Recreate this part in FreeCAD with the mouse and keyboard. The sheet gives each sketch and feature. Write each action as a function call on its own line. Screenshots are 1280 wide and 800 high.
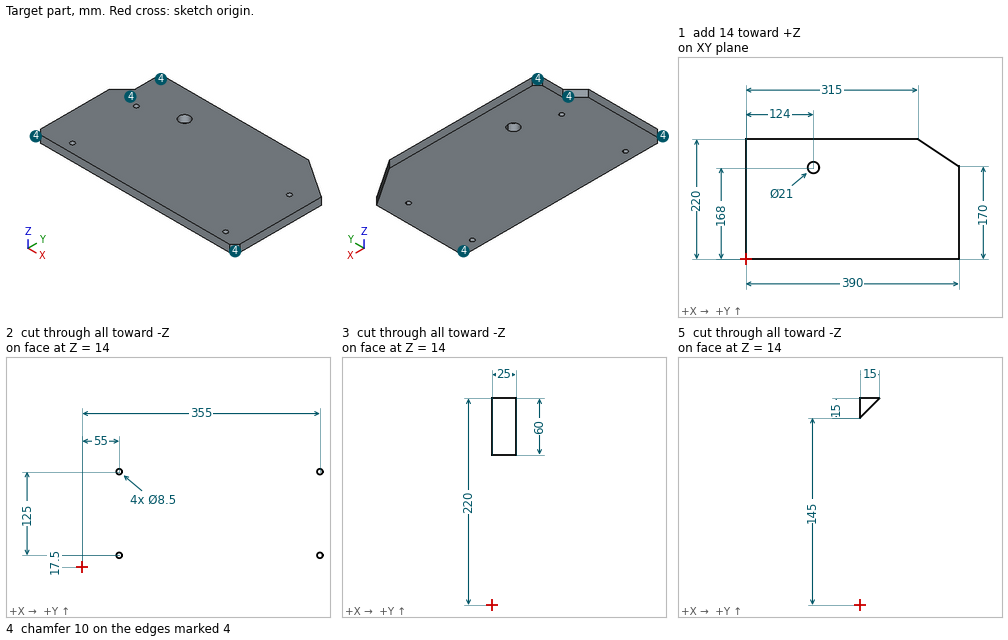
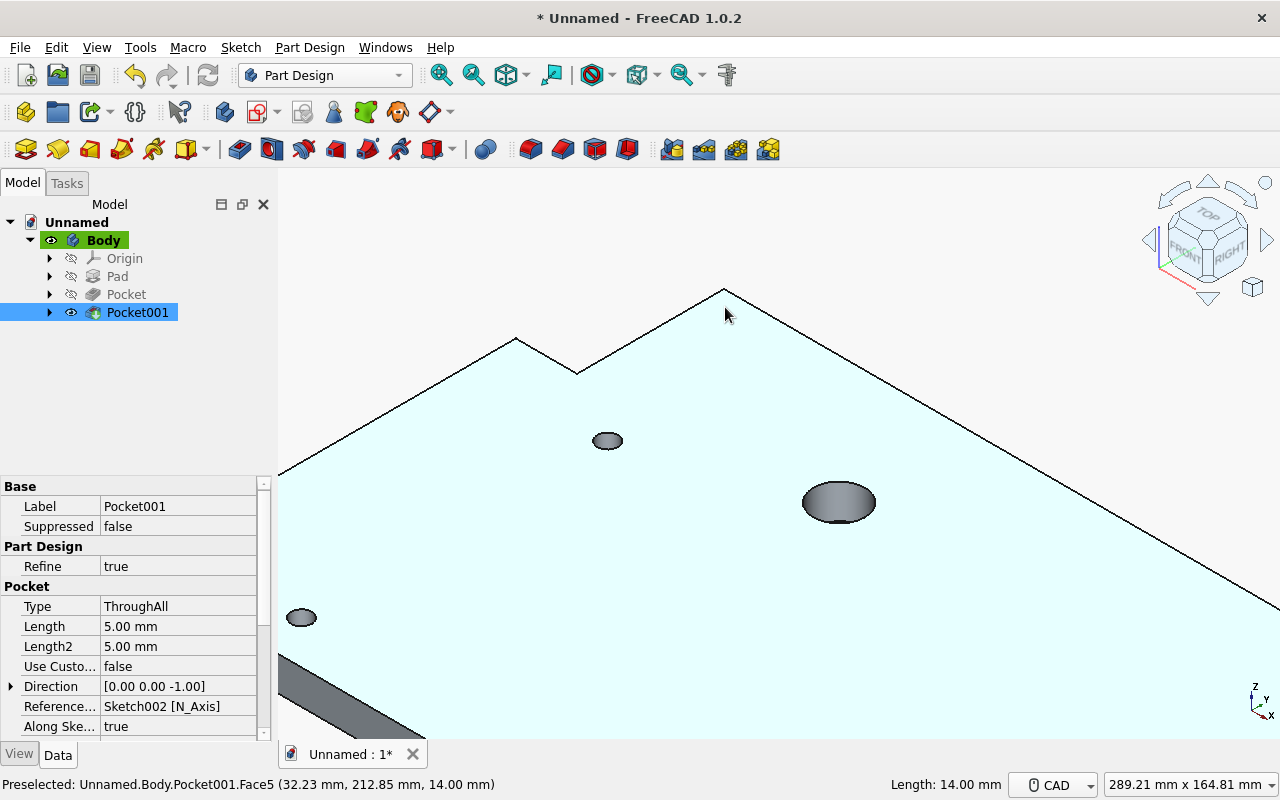
key(v)
key(f)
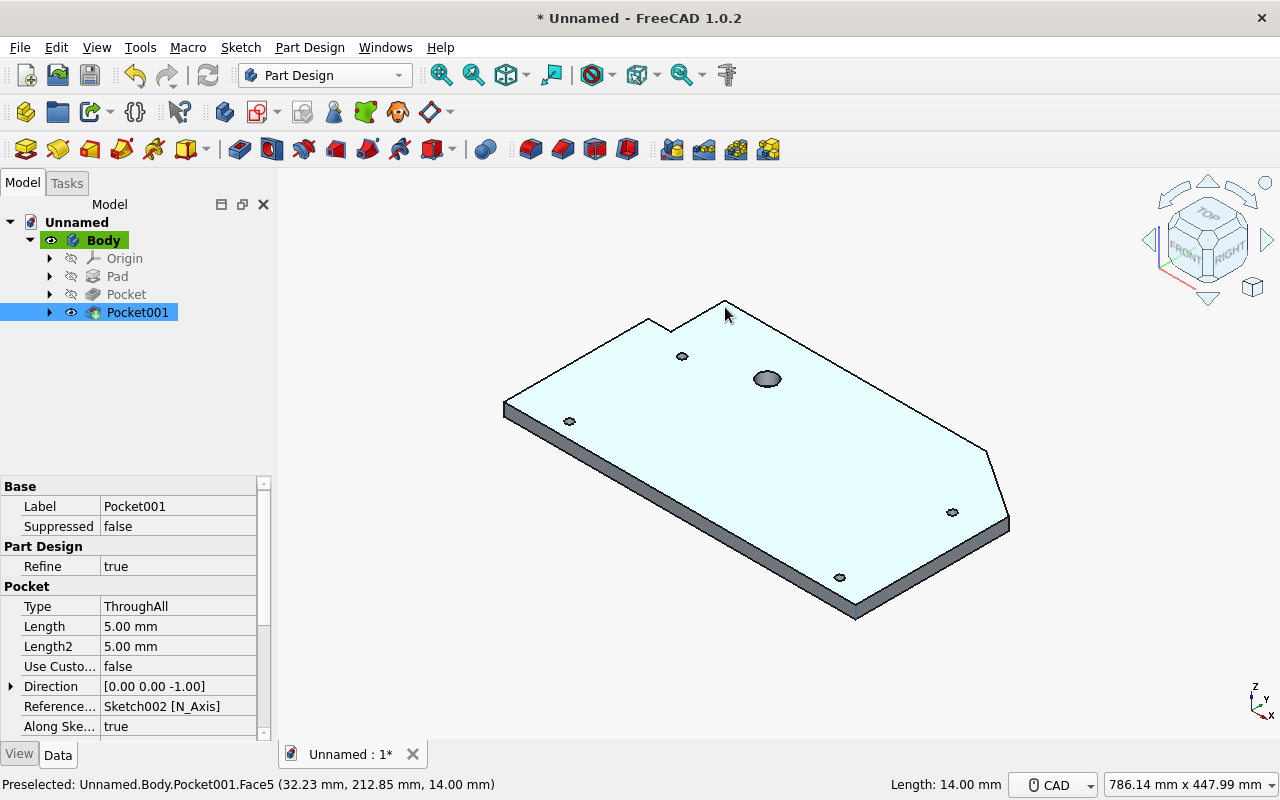
key(2)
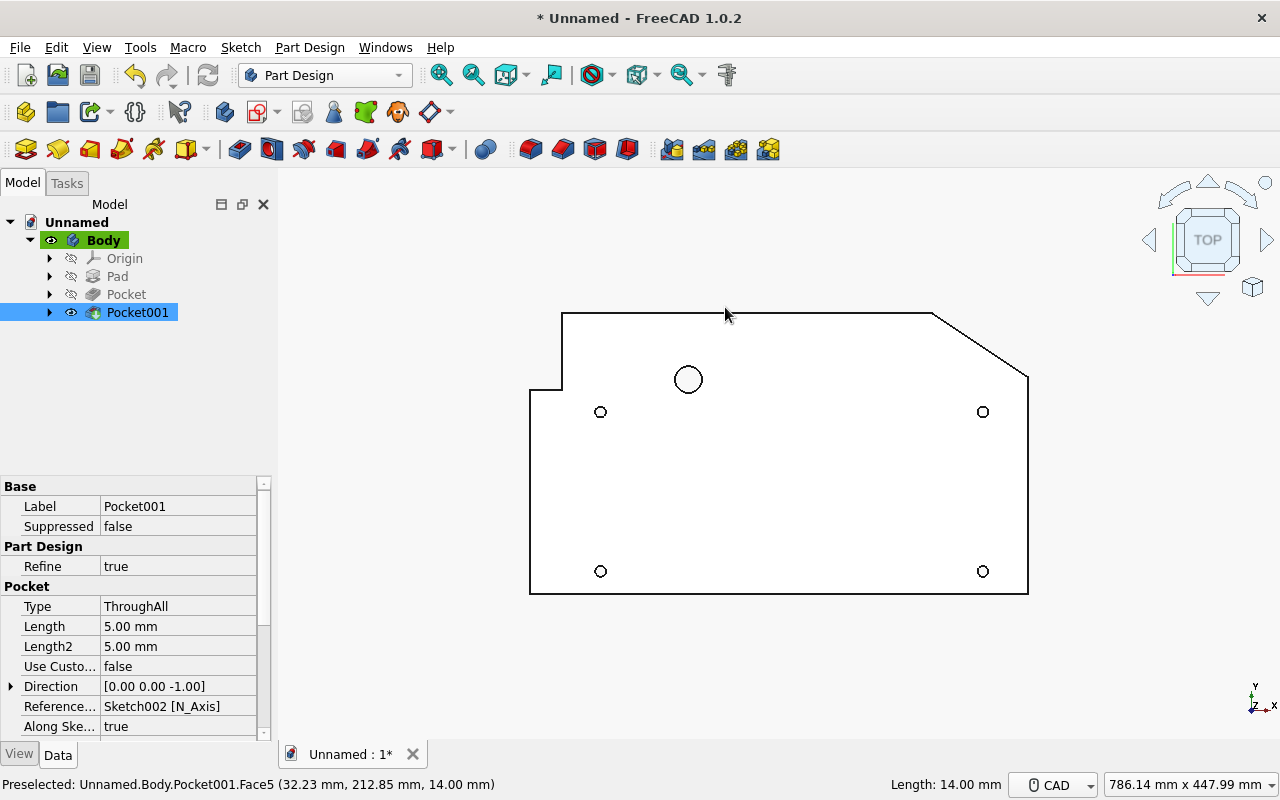
scroll(562, 312, up, 5)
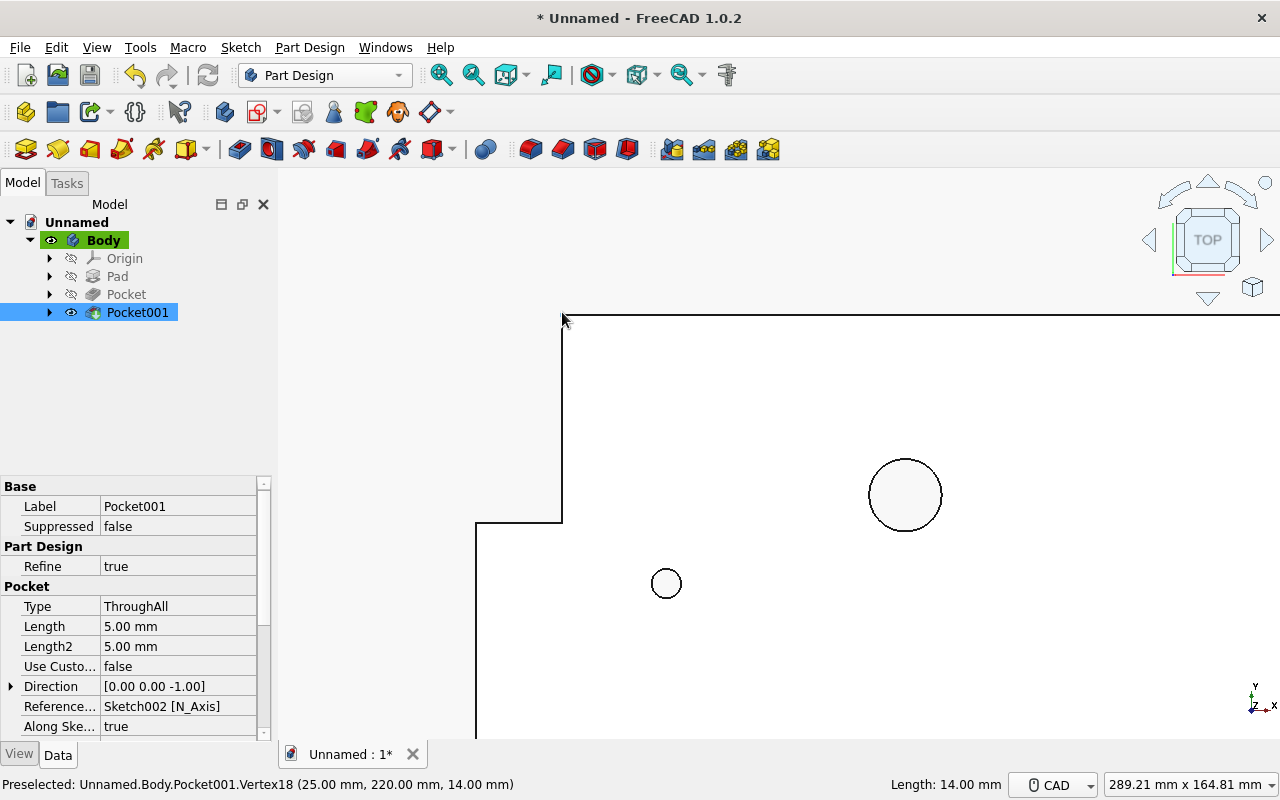
key(v)
key(f)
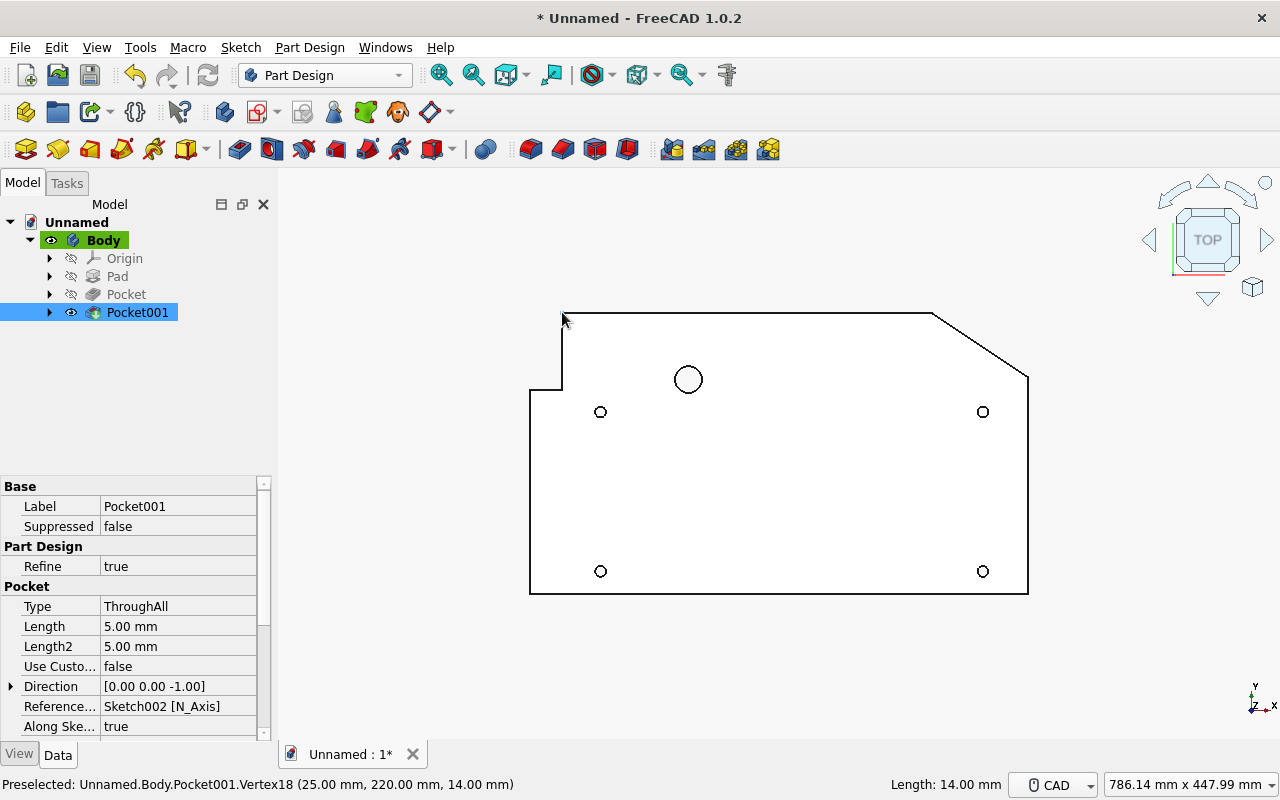
key(1)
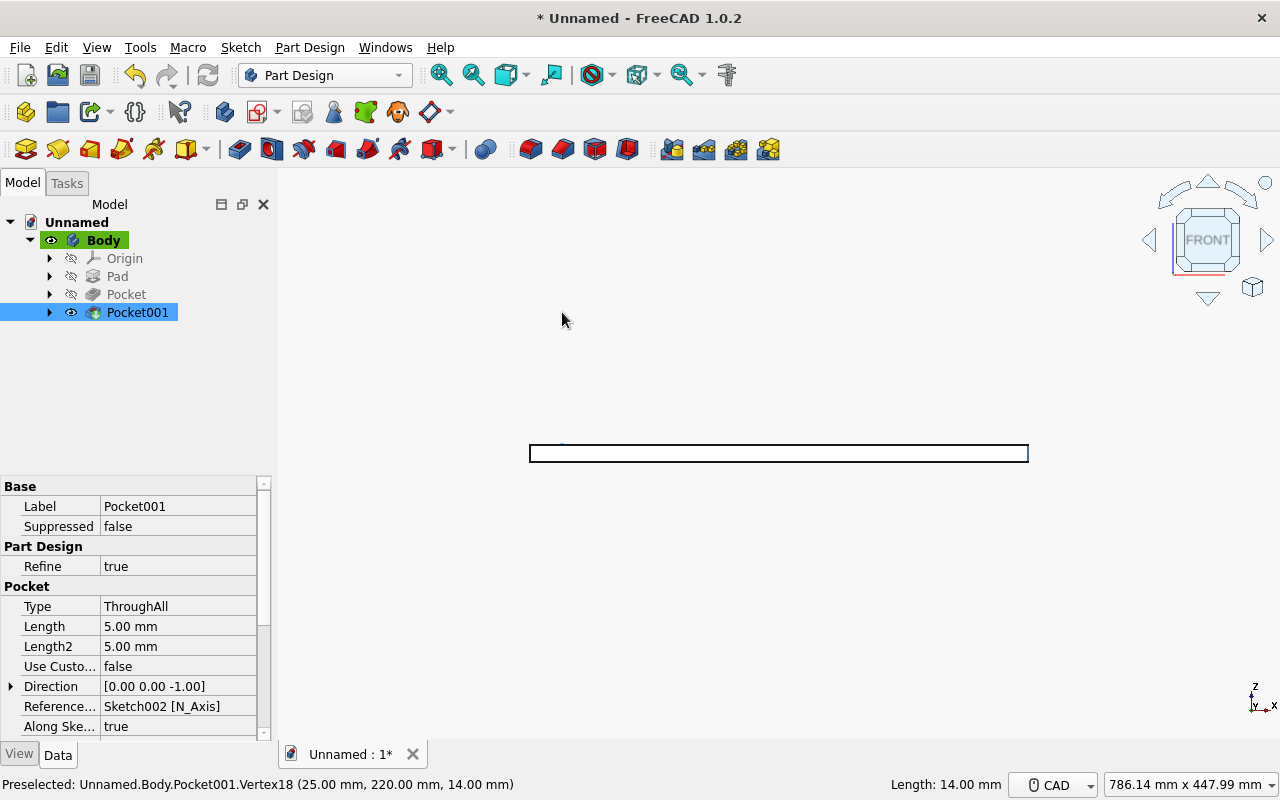
click(530, 453, ctrl)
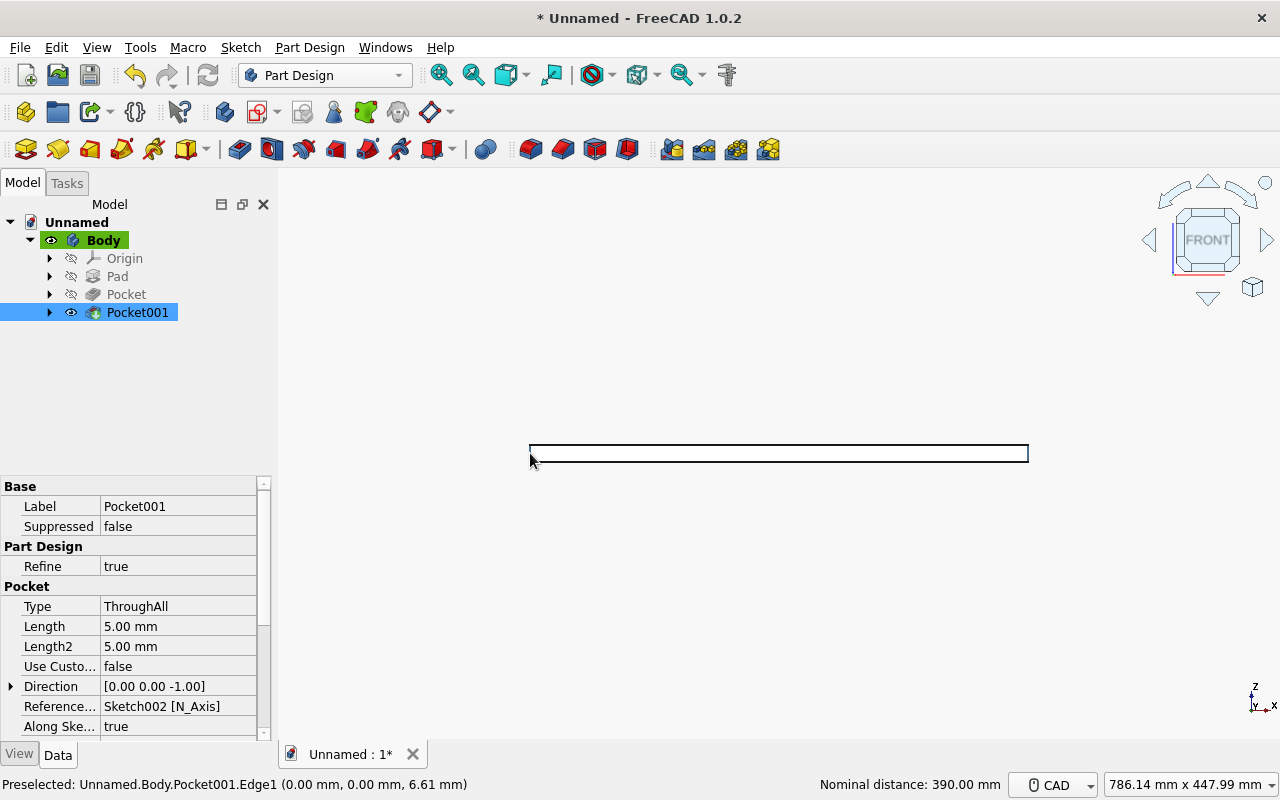
scroll(562, 453, up, 5)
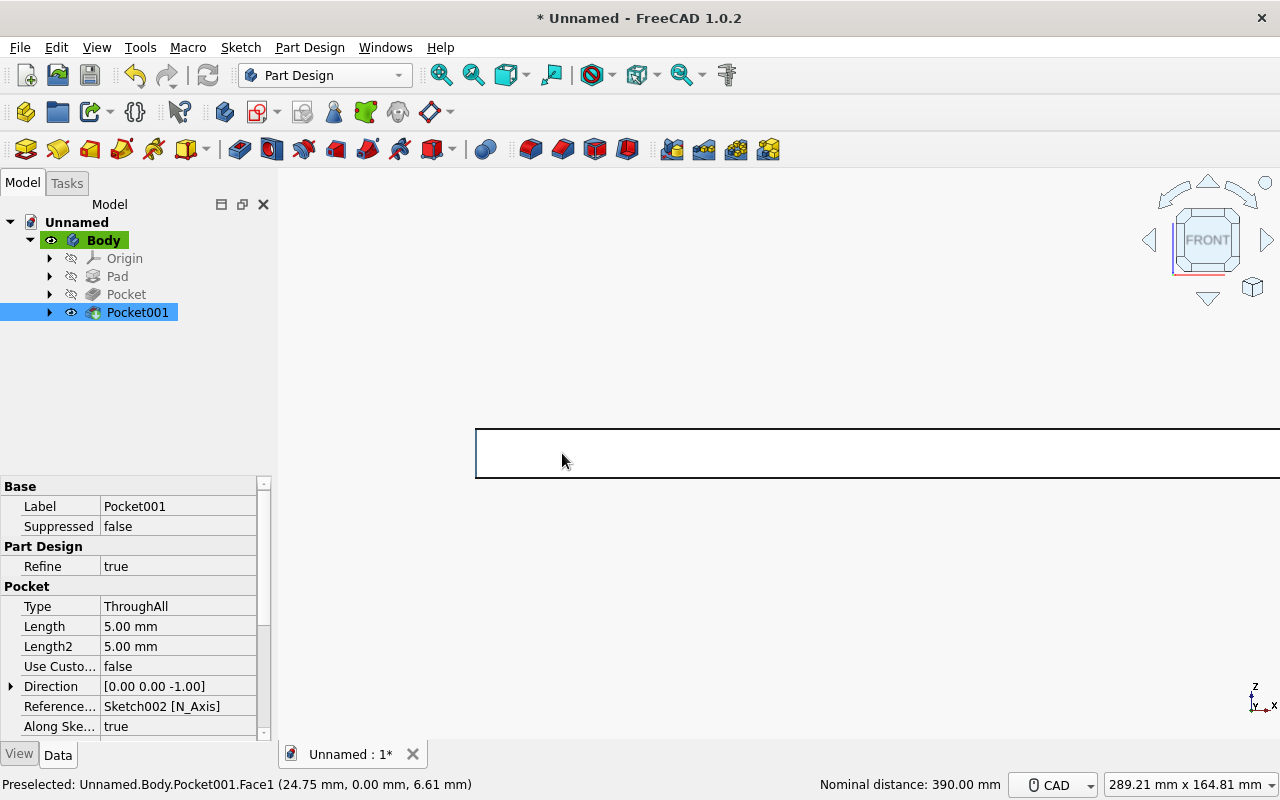
key(v)
key(f)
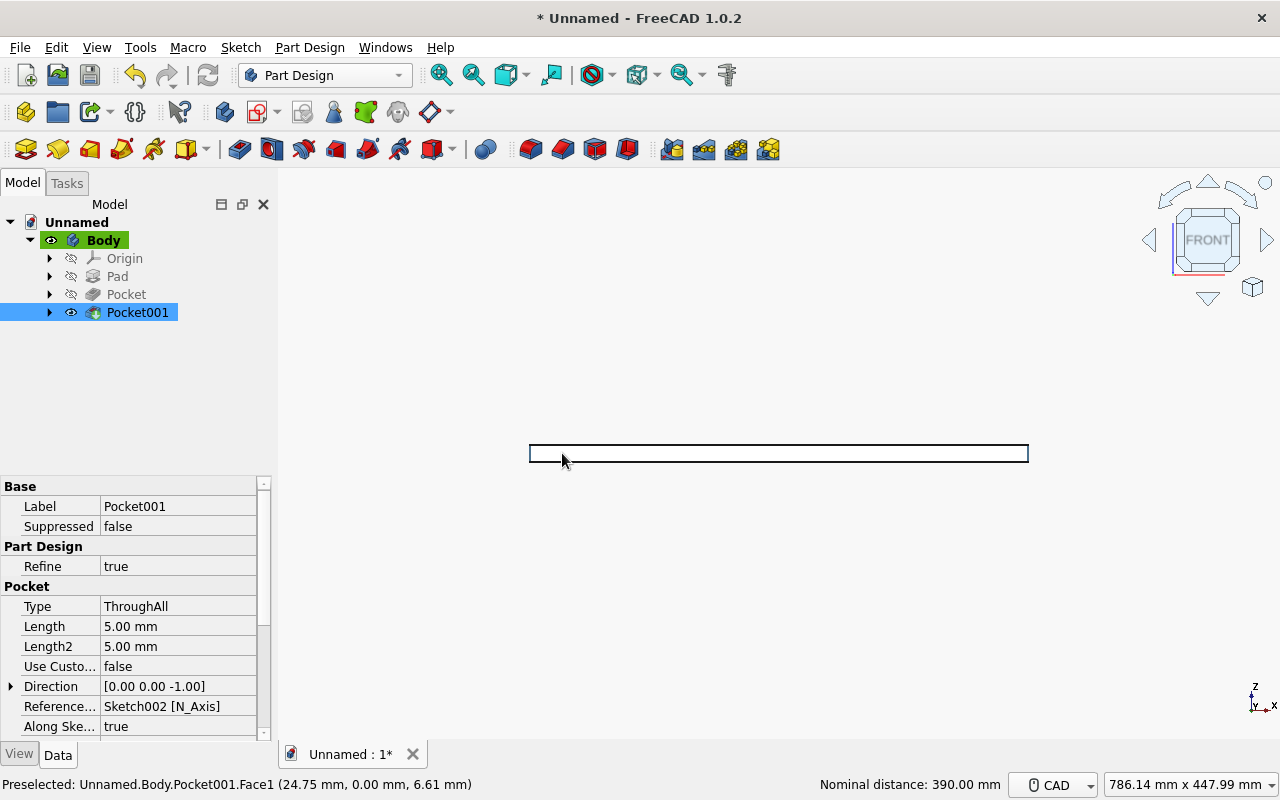
key(3)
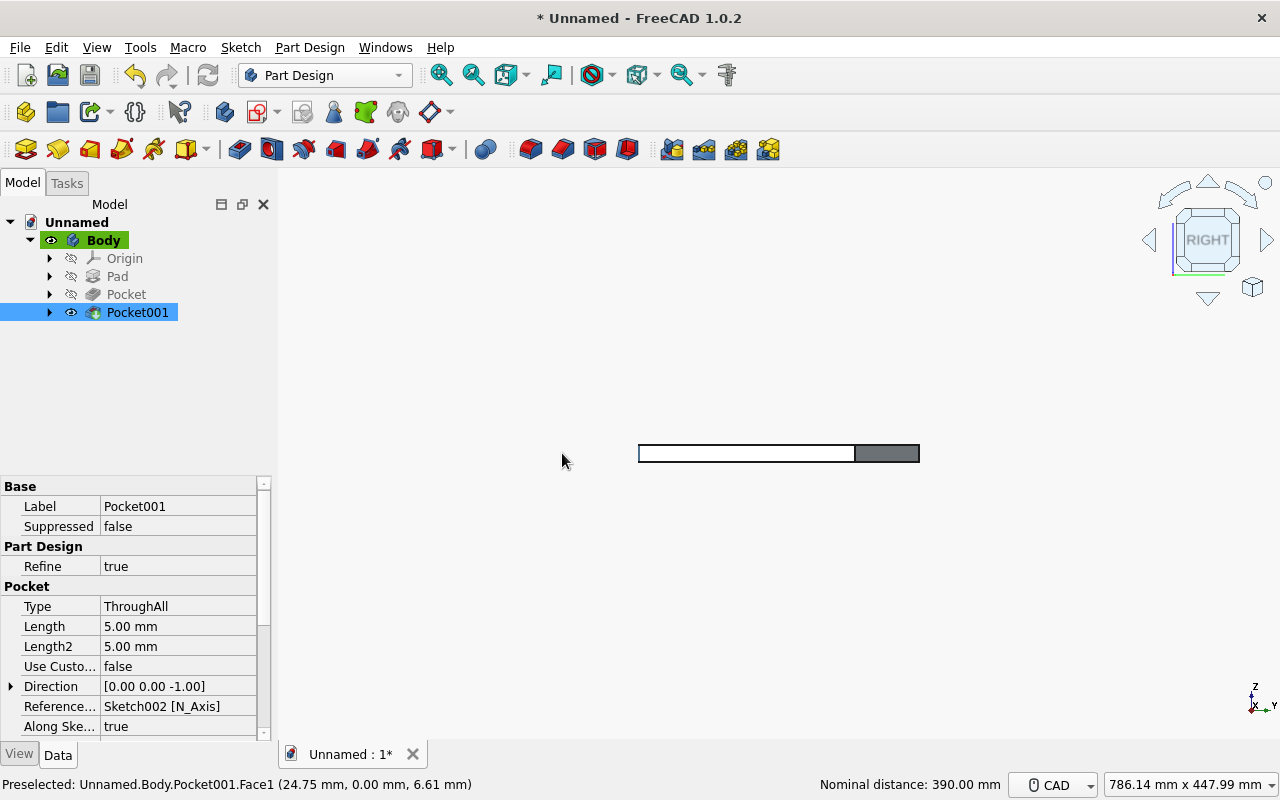
key(v)
key(f)